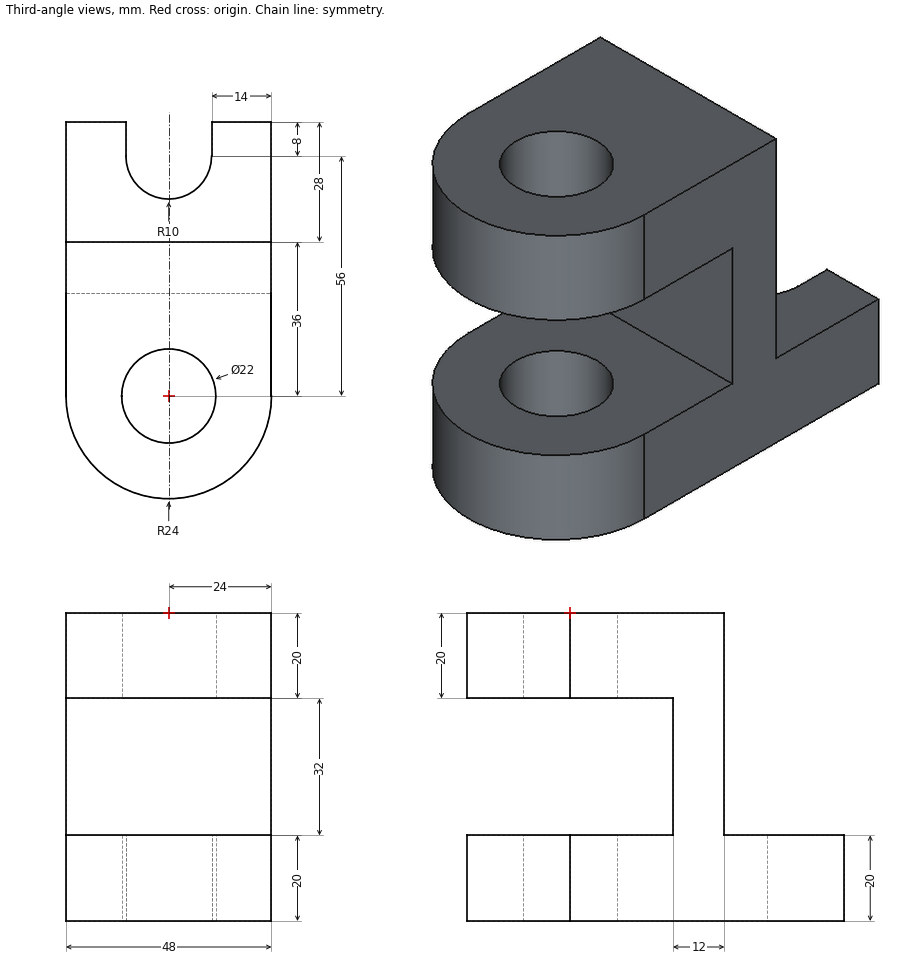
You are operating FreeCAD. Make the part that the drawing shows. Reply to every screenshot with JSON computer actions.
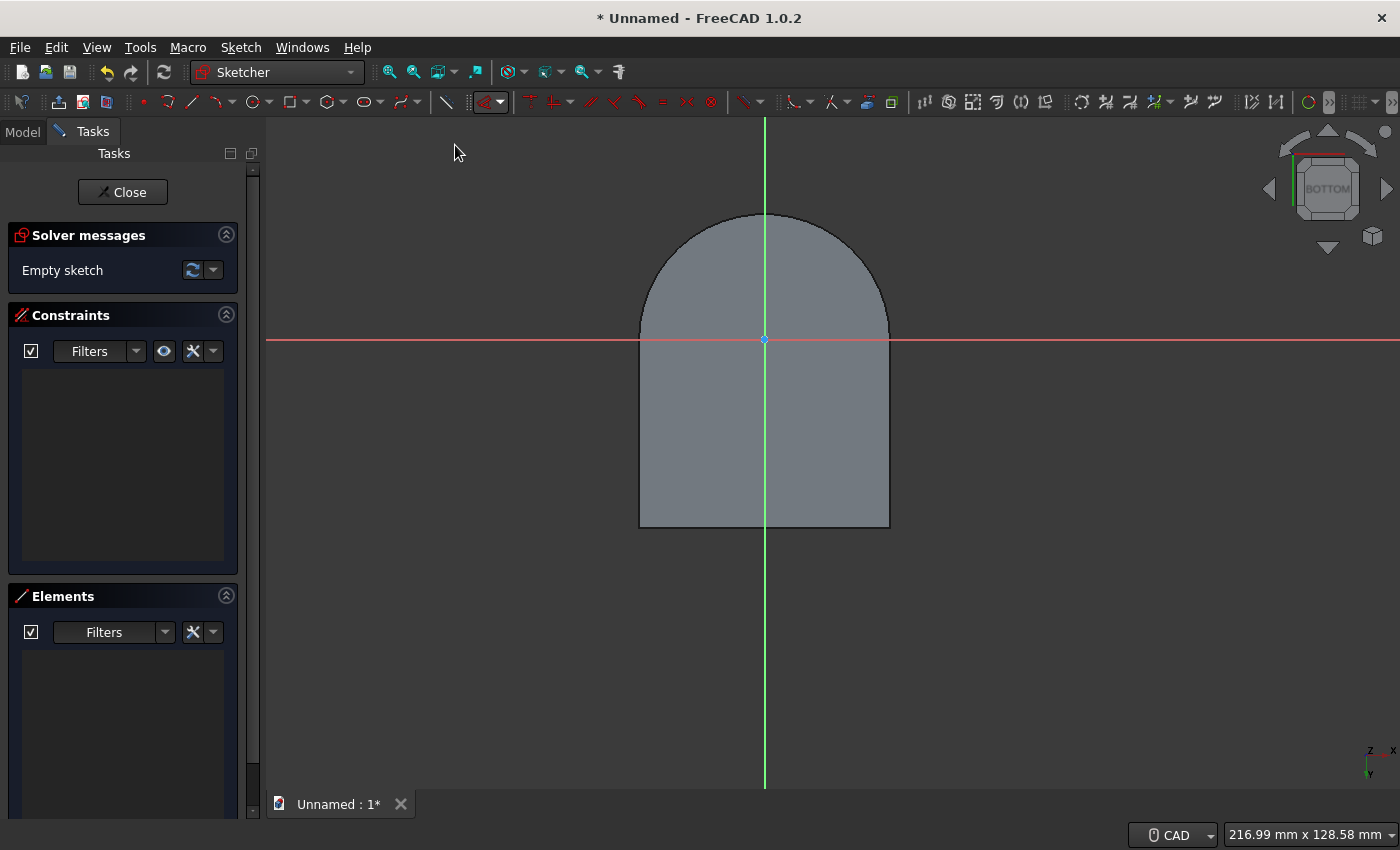
{"action": "left_click", "coordinate": [168, 102]}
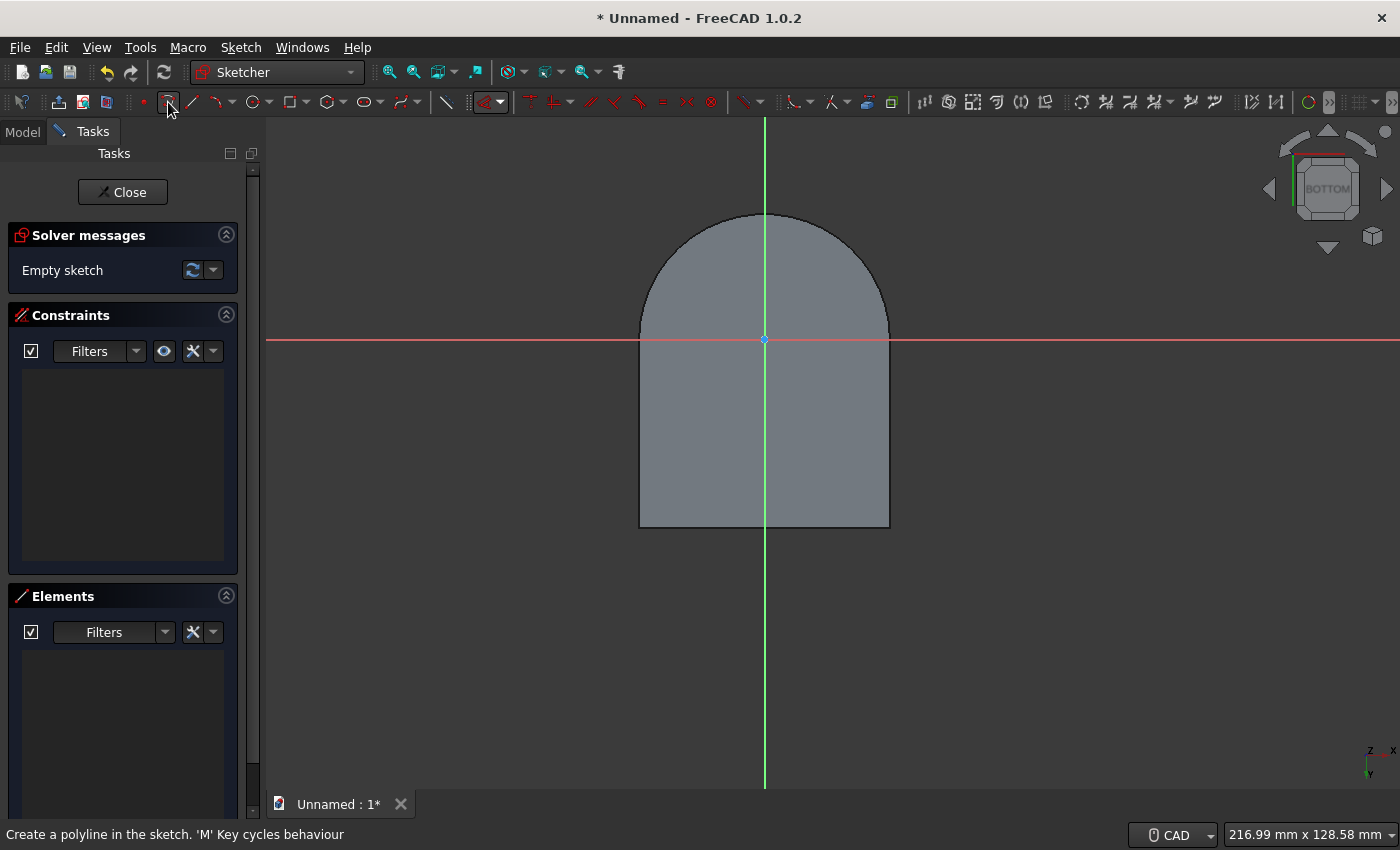
{"action": "left_click", "coordinate": [817, 632]}
{"action": "left_click", "coordinate": [817, 674]}
{"action": "left_click", "coordinate": [890, 674]}
{"action": "left_click", "coordinate": [890, 528]}
{"action": "left_click", "coordinate": [639, 528]}
{"action": "left_click", "coordinate": [639, 674]}
{"action": "left_click", "coordinate": [712, 674]}
{"action": "left_click", "coordinate": [712, 632]}
{"action": "right_click", "coordinate": [712, 632]}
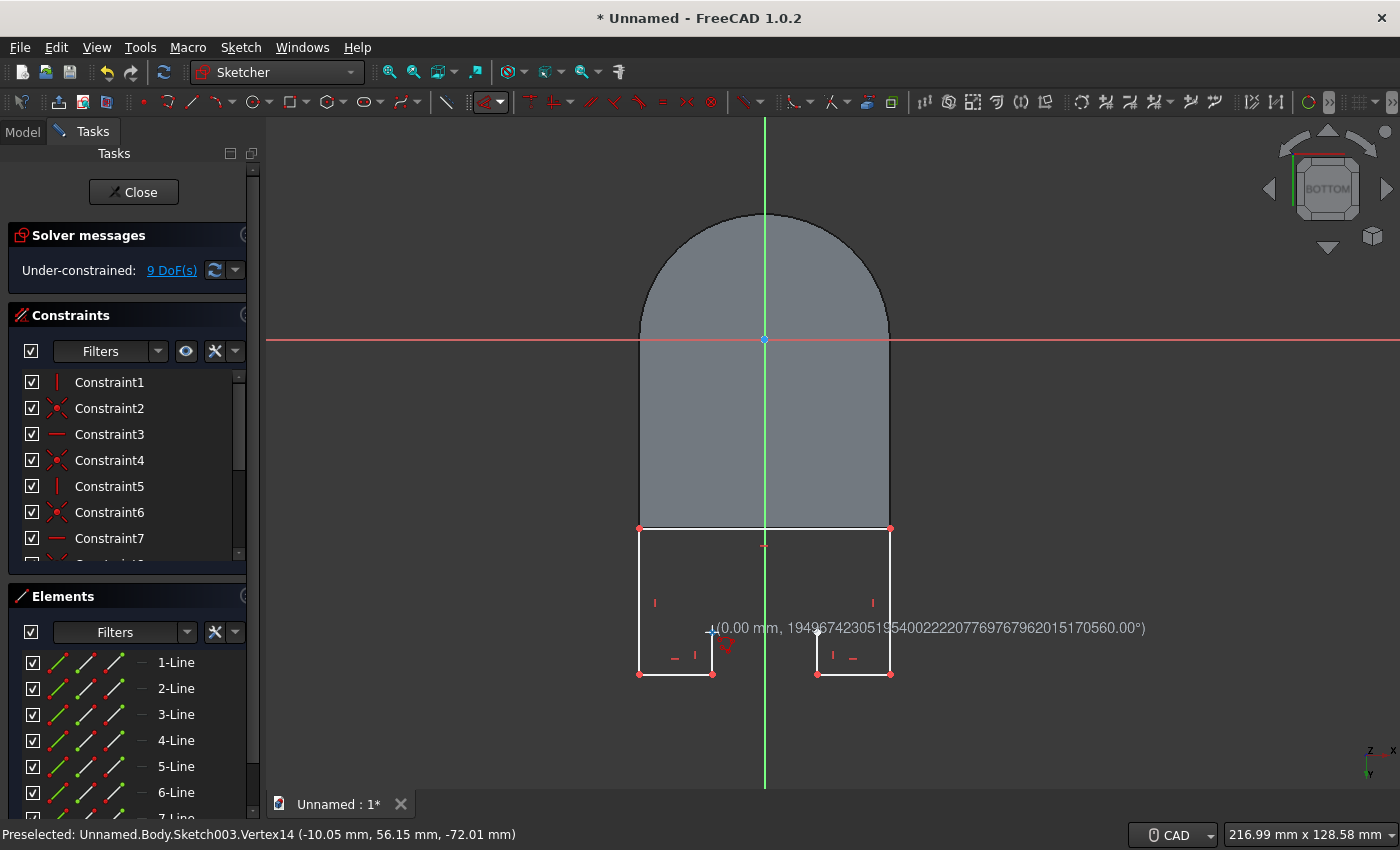
{"action": "left_click", "coordinate": [216, 102]}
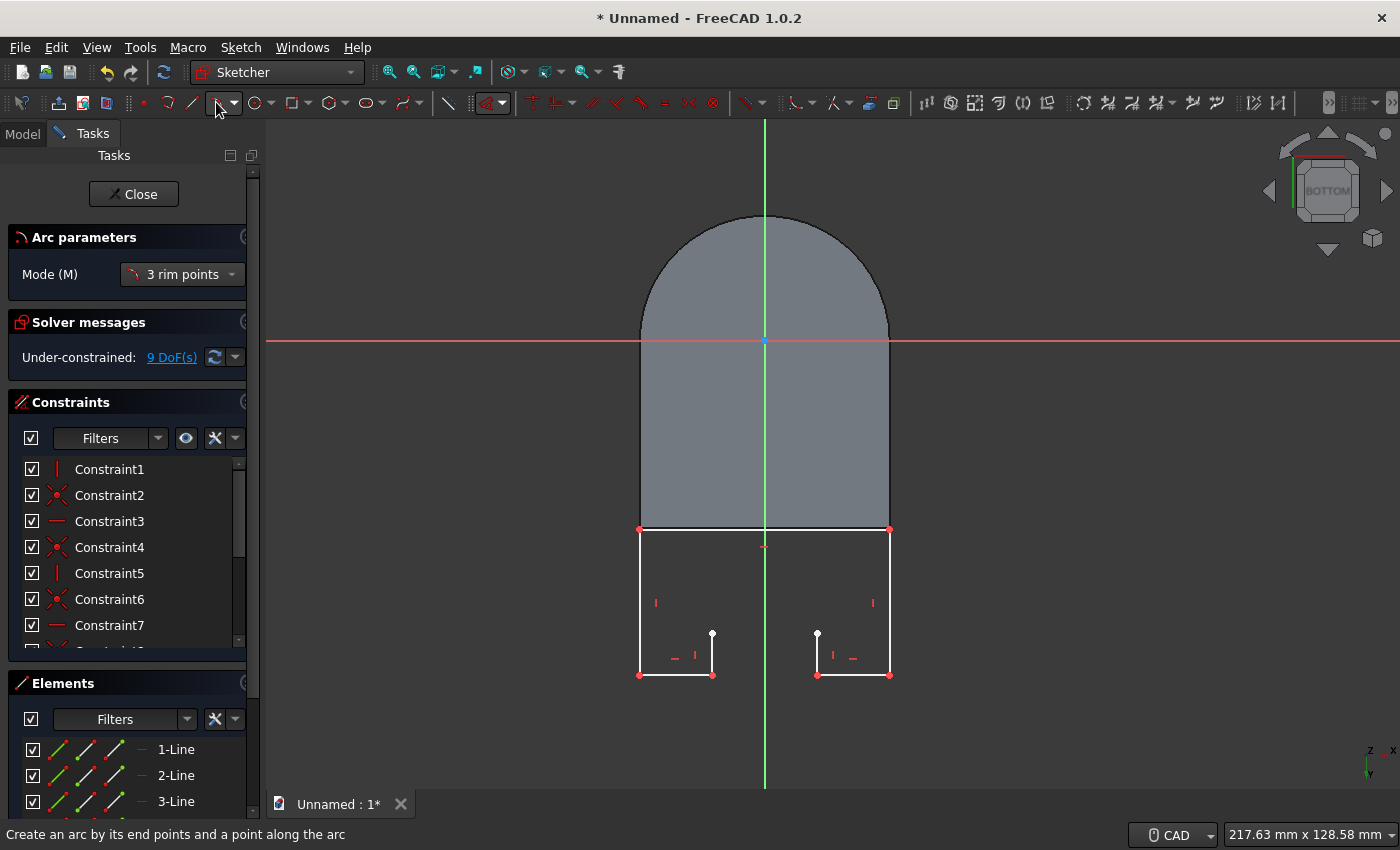
{"action": "left_click", "coordinate": [712, 633]}
{"action": "left_click", "coordinate": [817, 633]}
{"action": "left_click", "coordinate": [781, 583]}
{"action": "key", "text": "Escape"}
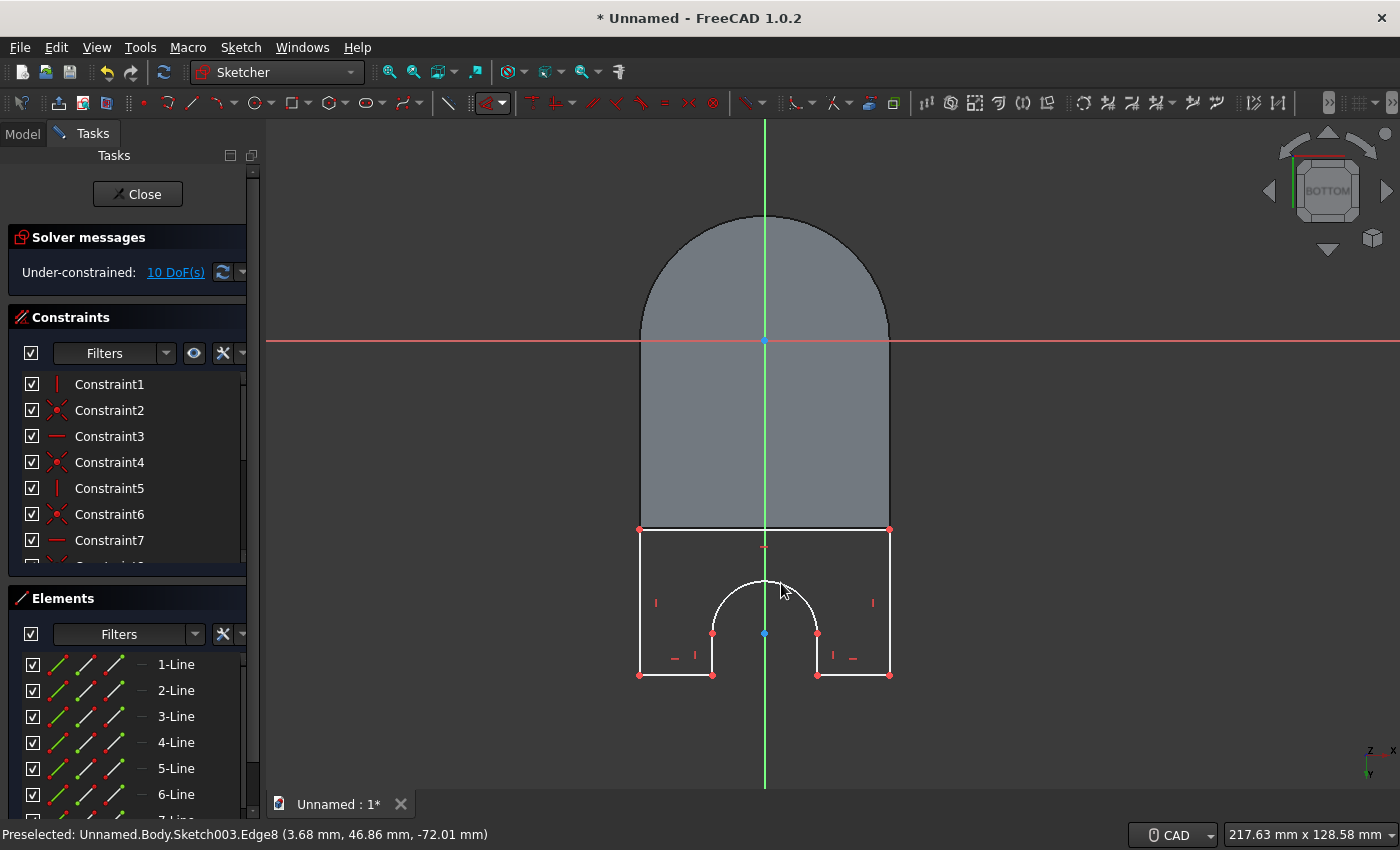
{"action": "left_click", "coordinate": [817, 646]}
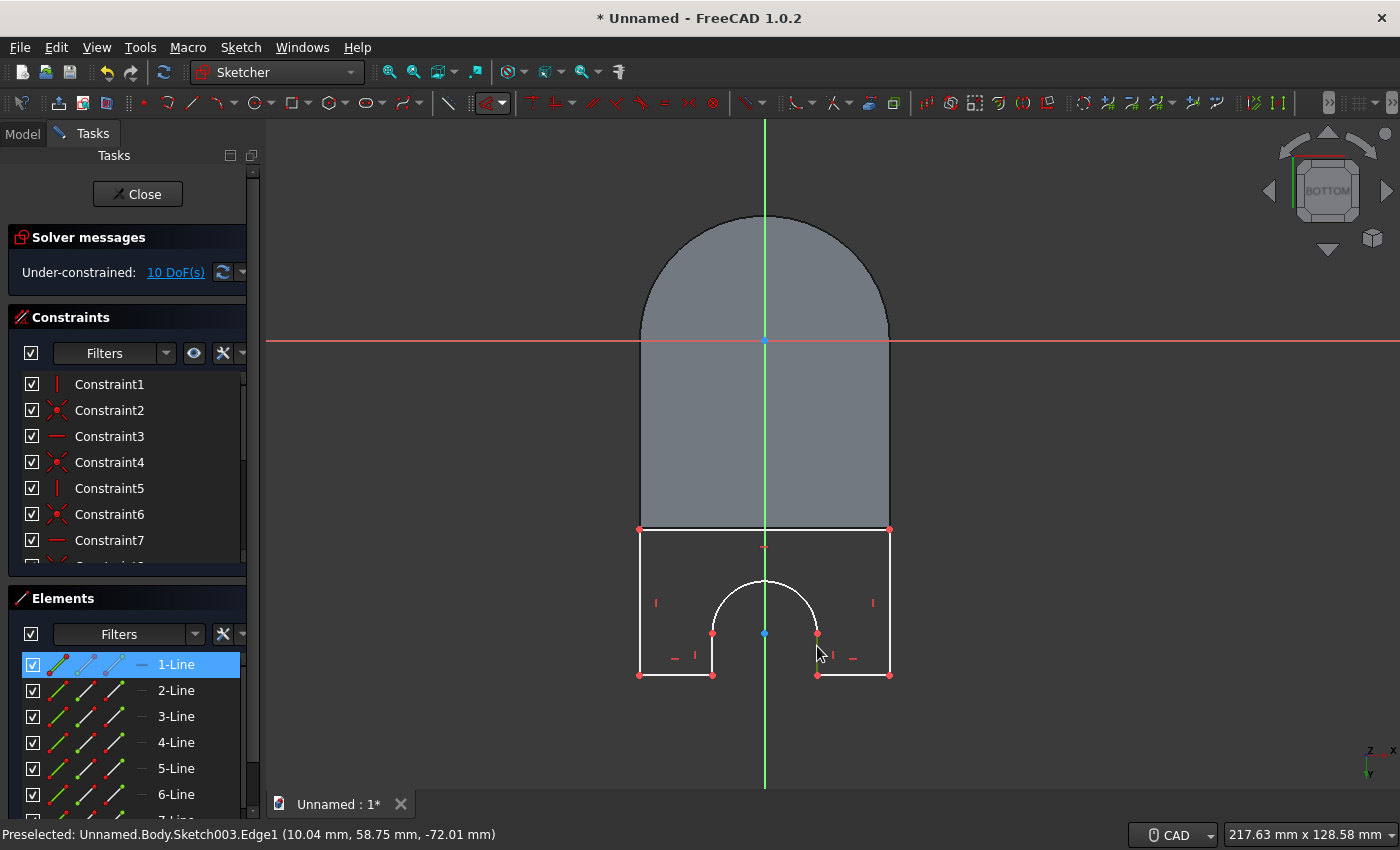
{"action": "left_click", "coordinate": [795, 591]}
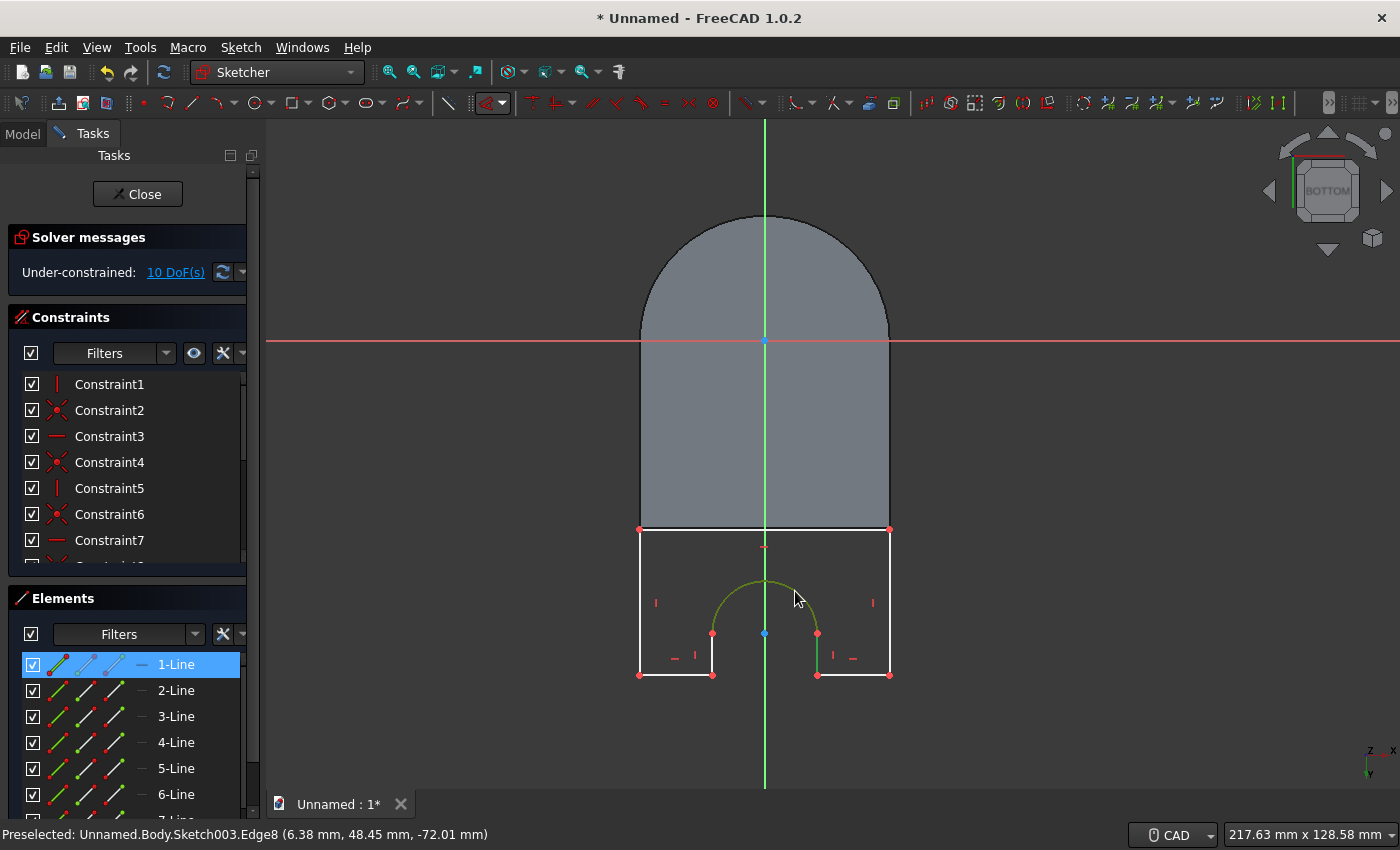
{"action": "left_click", "coordinate": [642, 104]}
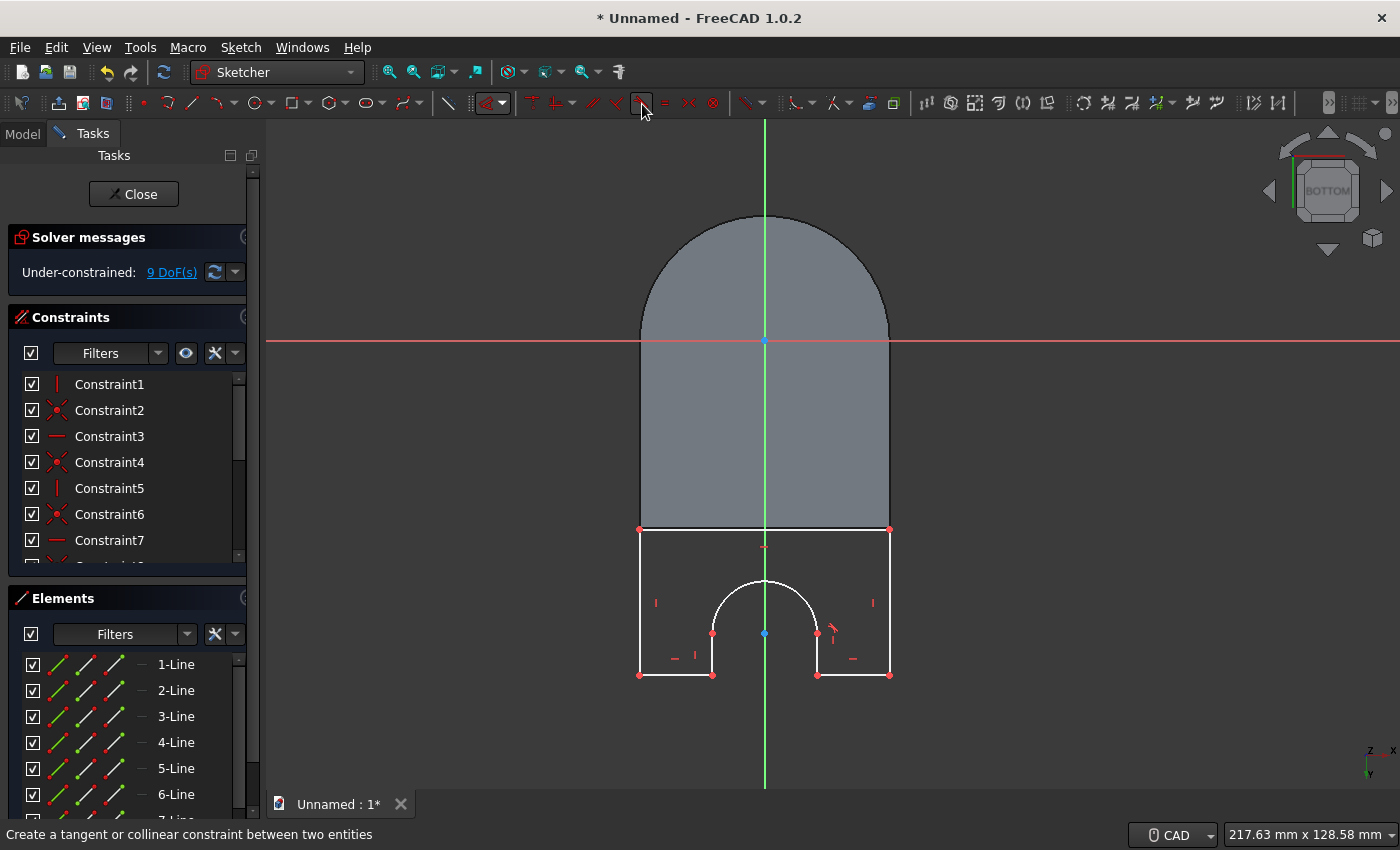
{"action": "left_click", "coordinate": [712, 663]}